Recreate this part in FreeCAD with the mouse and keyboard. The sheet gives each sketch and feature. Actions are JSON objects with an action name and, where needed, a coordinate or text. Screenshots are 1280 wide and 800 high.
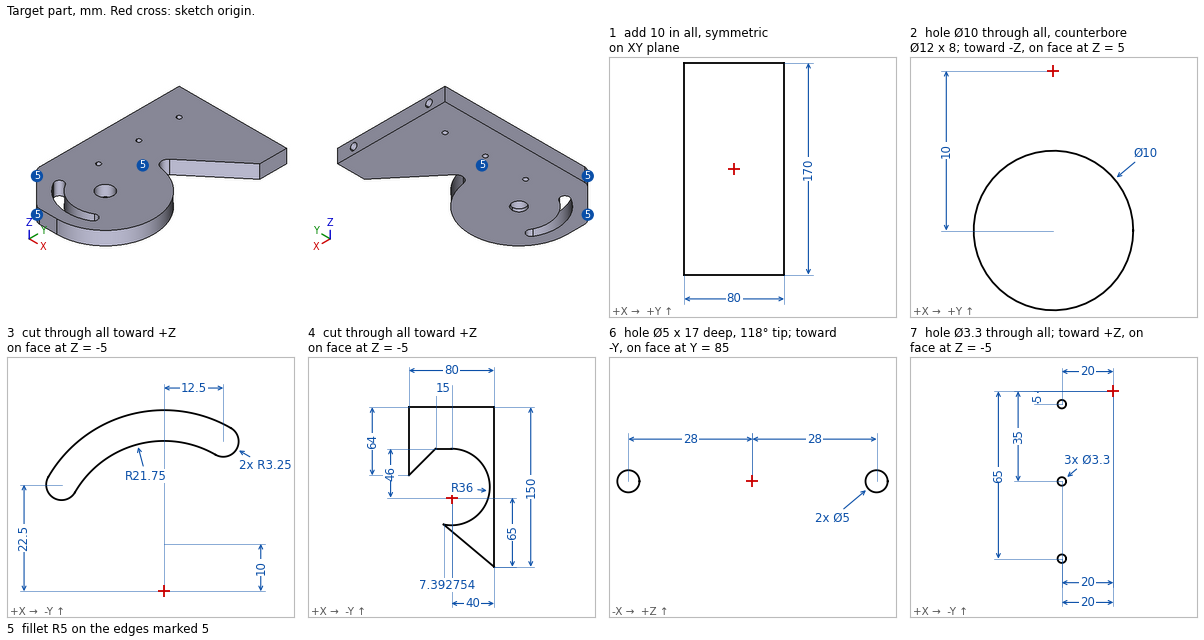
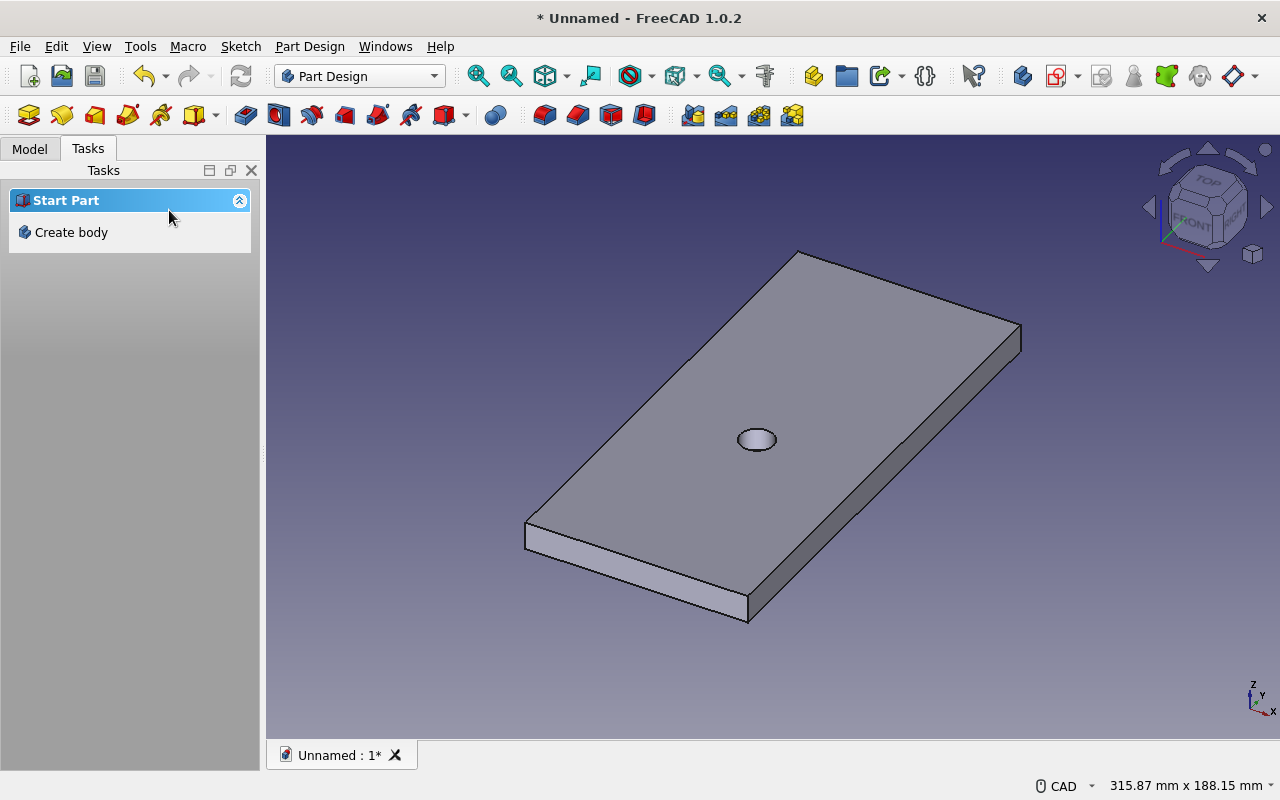
{"action": "key", "text": "5"}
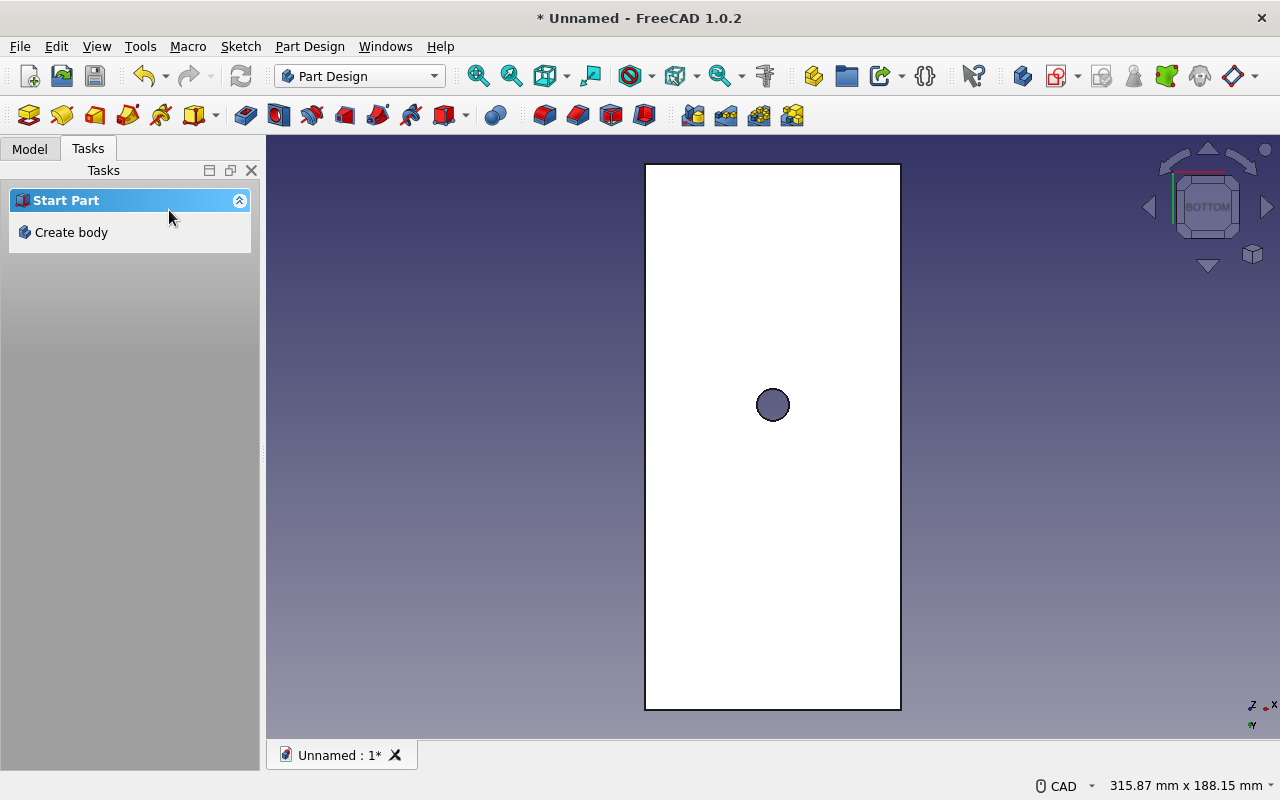
{"action": "left_click", "coordinate": [773, 592]}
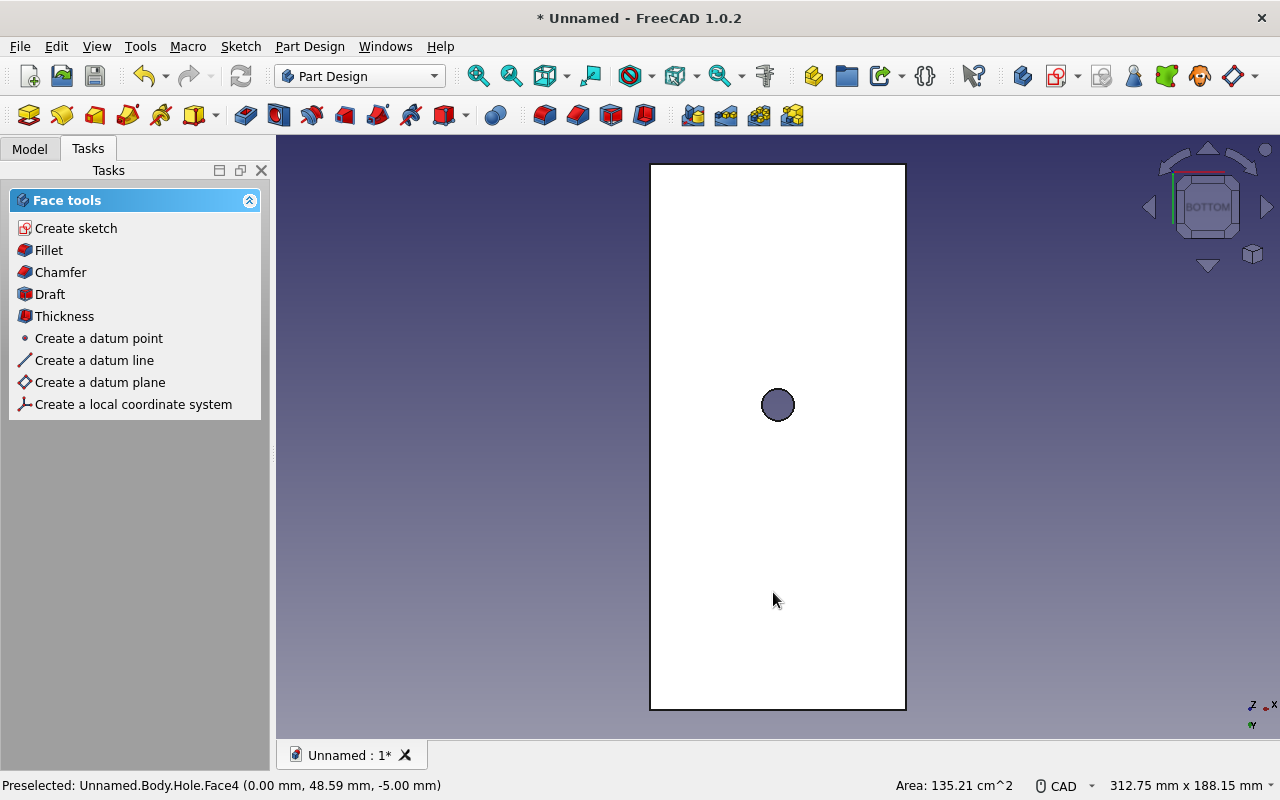
{"action": "left_click", "coordinate": [1056, 76]}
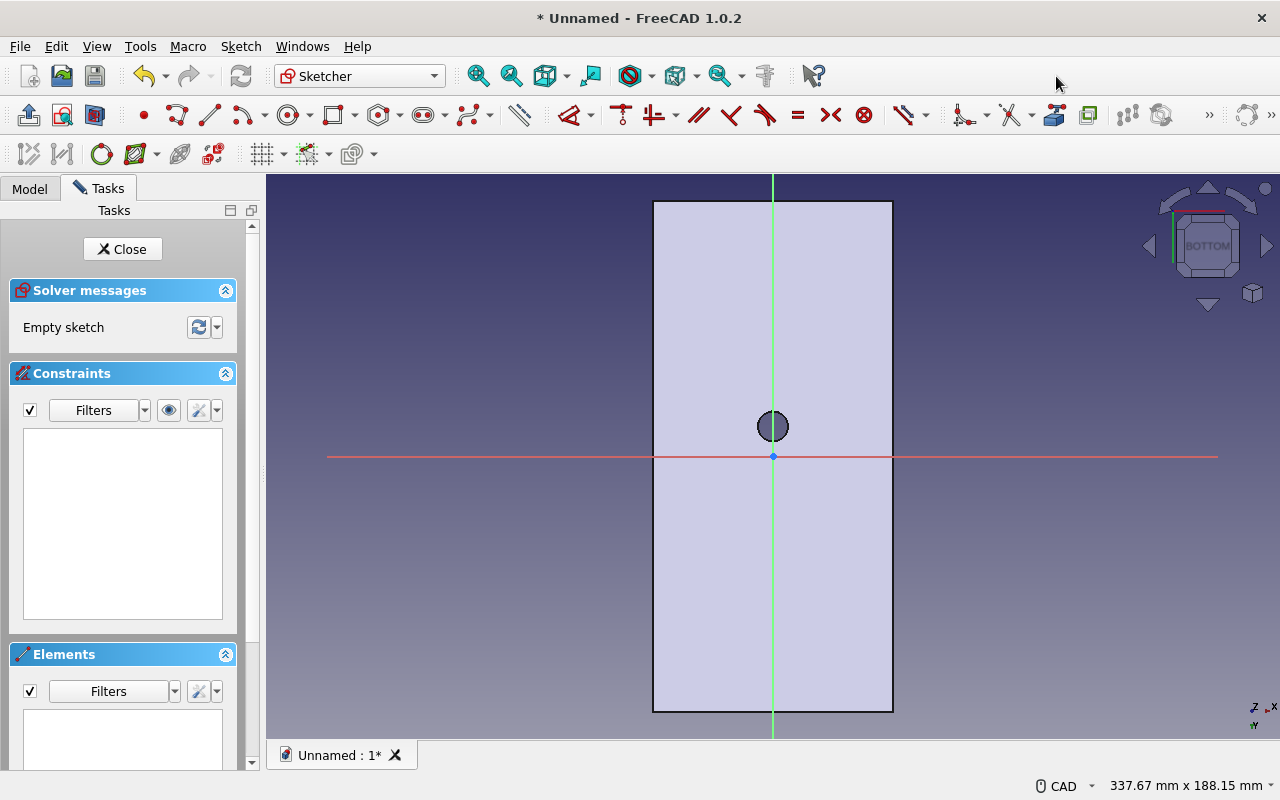
{"action": "scroll", "coordinate": [783, 376], "scroll_direction": "up", "scroll_amount": 6}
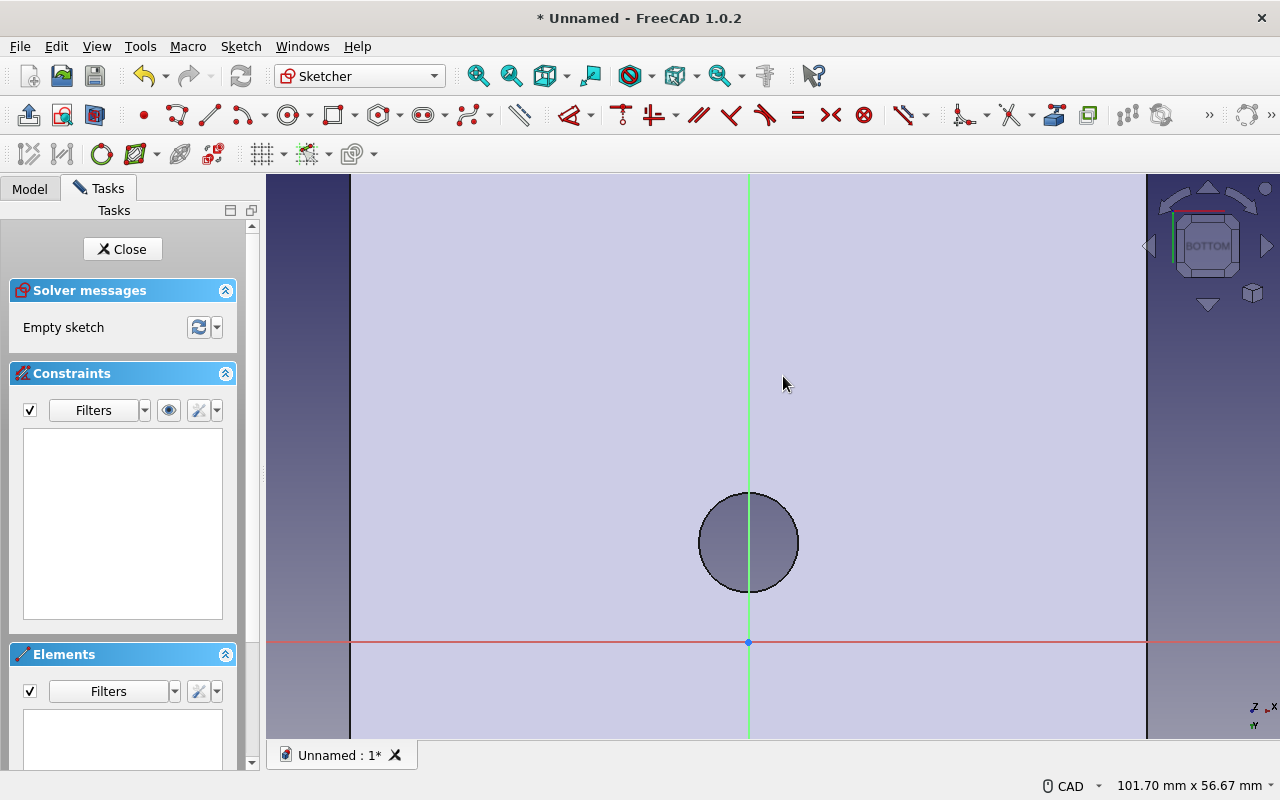
{"action": "key", "text": "g 3 a"}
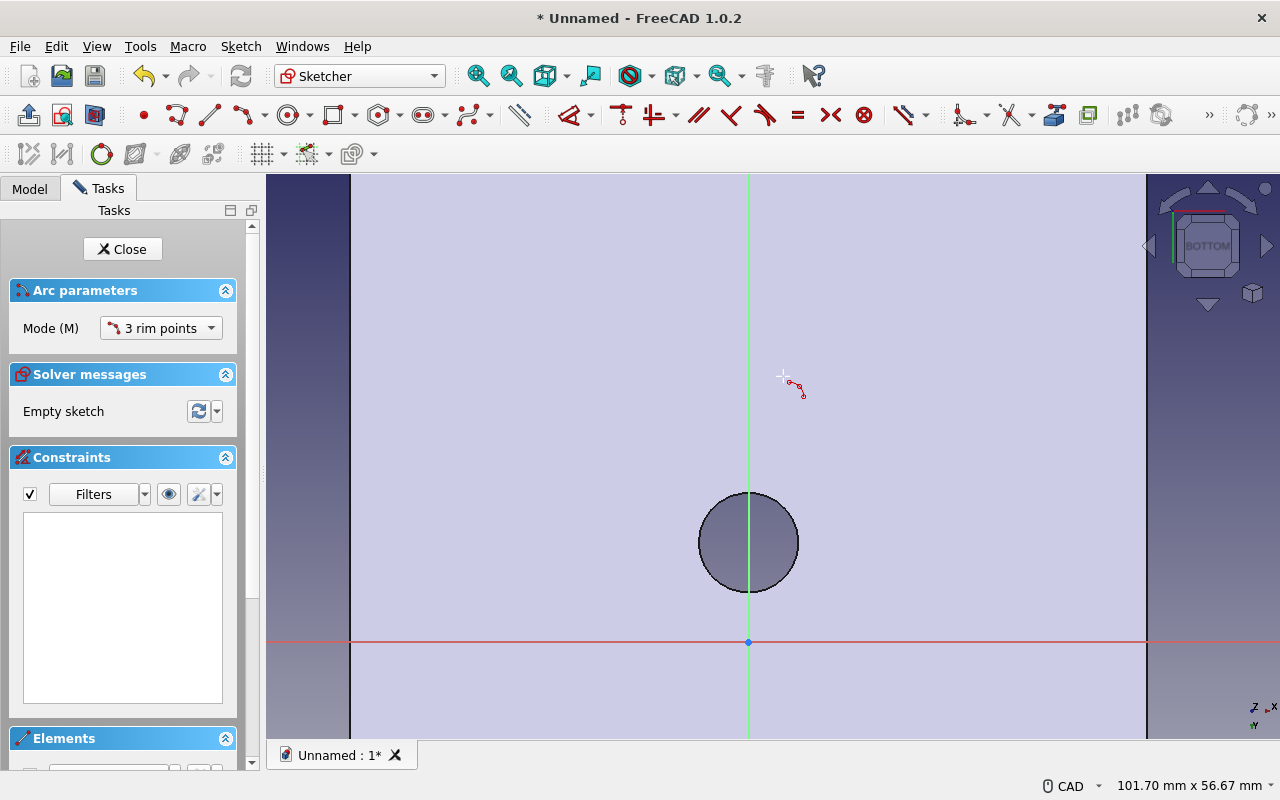
{"action": "left_click", "coordinate": [561, 434]}
{"action": "left_click", "coordinate": [857, 355]}
{"action": "left_click", "coordinate": [692, 333]}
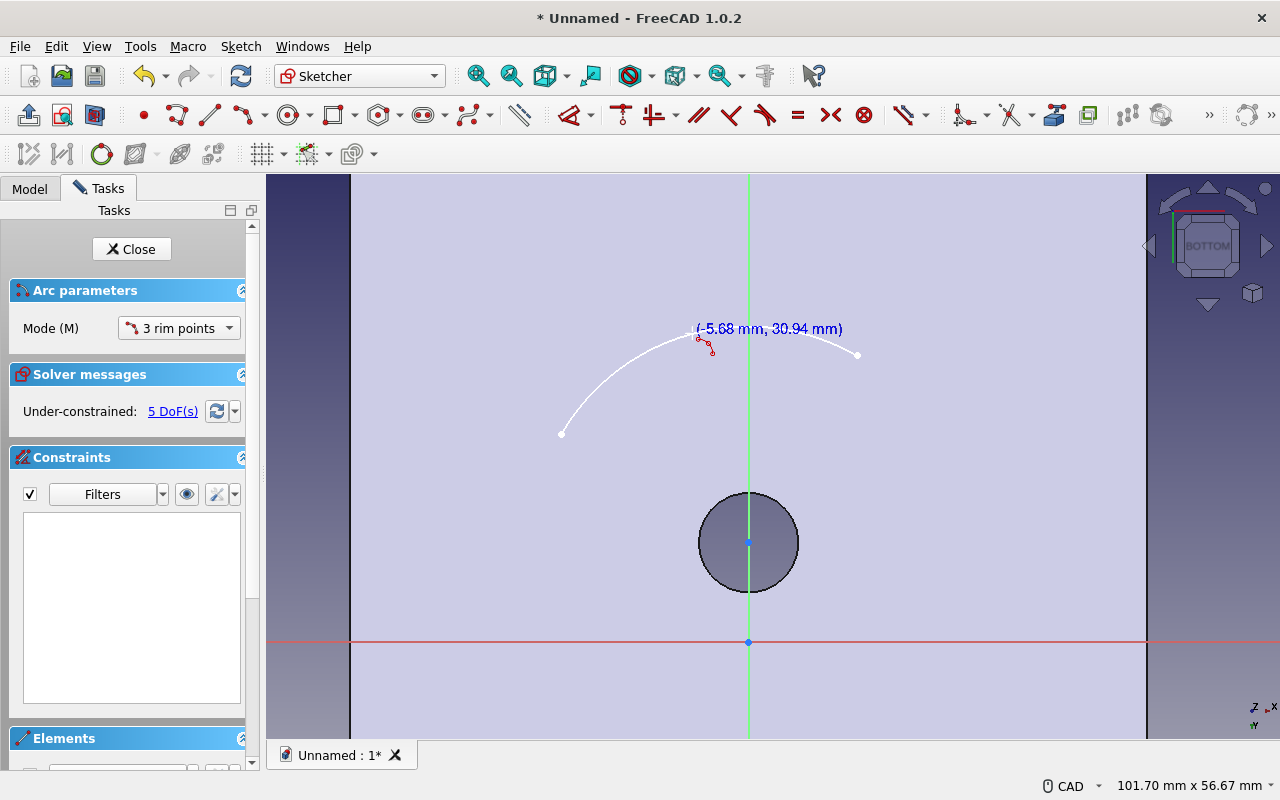
{"action": "left_click", "coordinate": [857, 356]}
{"action": "left_click", "coordinate": [889, 299]}
{"action": "left_click", "coordinate": [901, 343]}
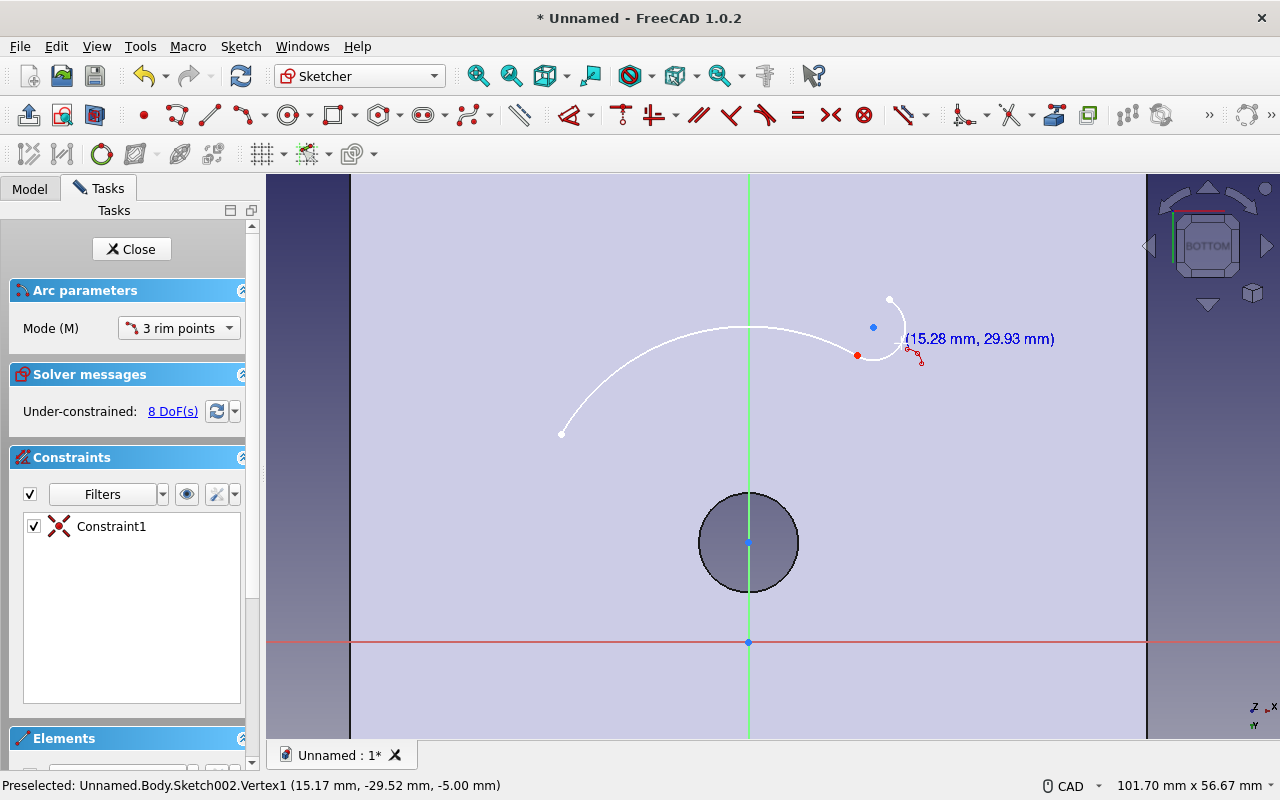
{"action": "left_click", "coordinate": [889, 300]}
{"action": "left_click", "coordinate": [505, 402]}
{"action": "left_click", "coordinate": [676, 271]}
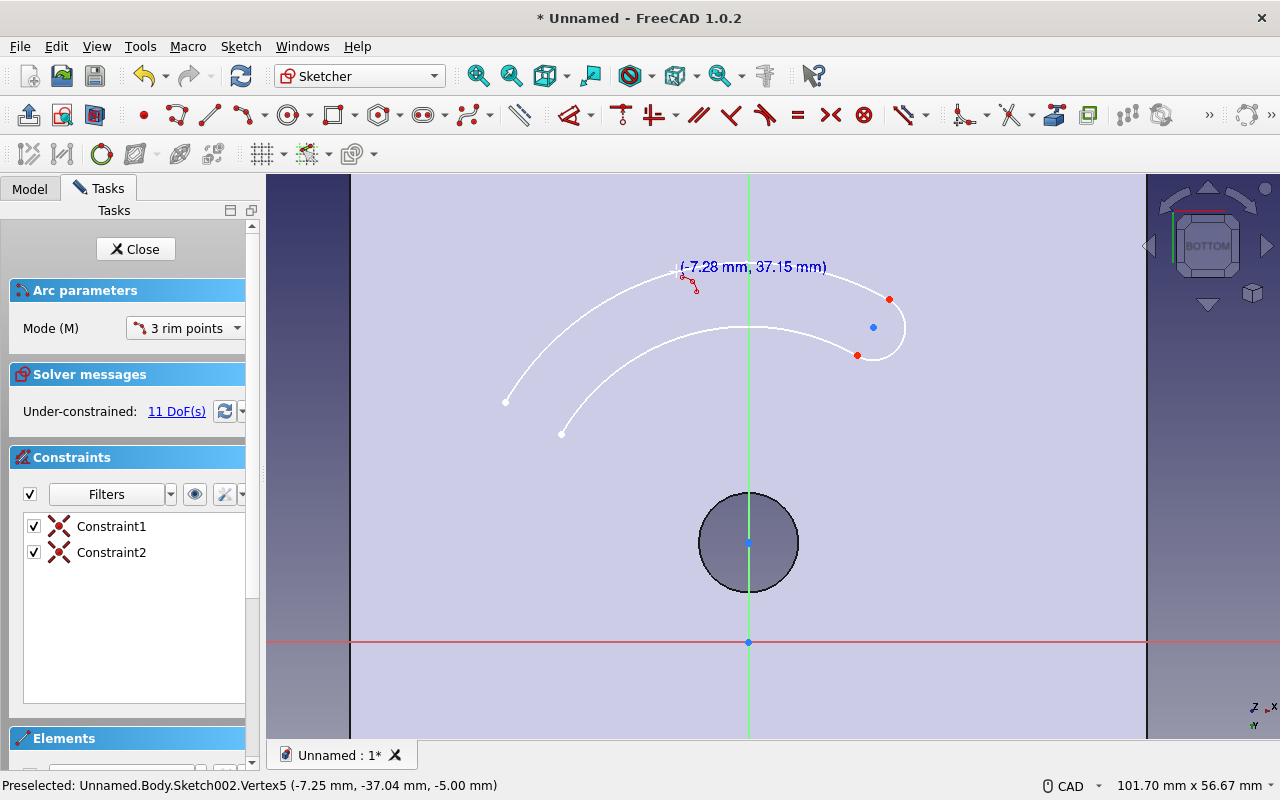
{"action": "left_click", "coordinate": [505, 403]}
{"action": "left_click", "coordinate": [561, 435]}
{"action": "left_click", "coordinate": [517, 446]}
{"action": "key", "text": "Escape"}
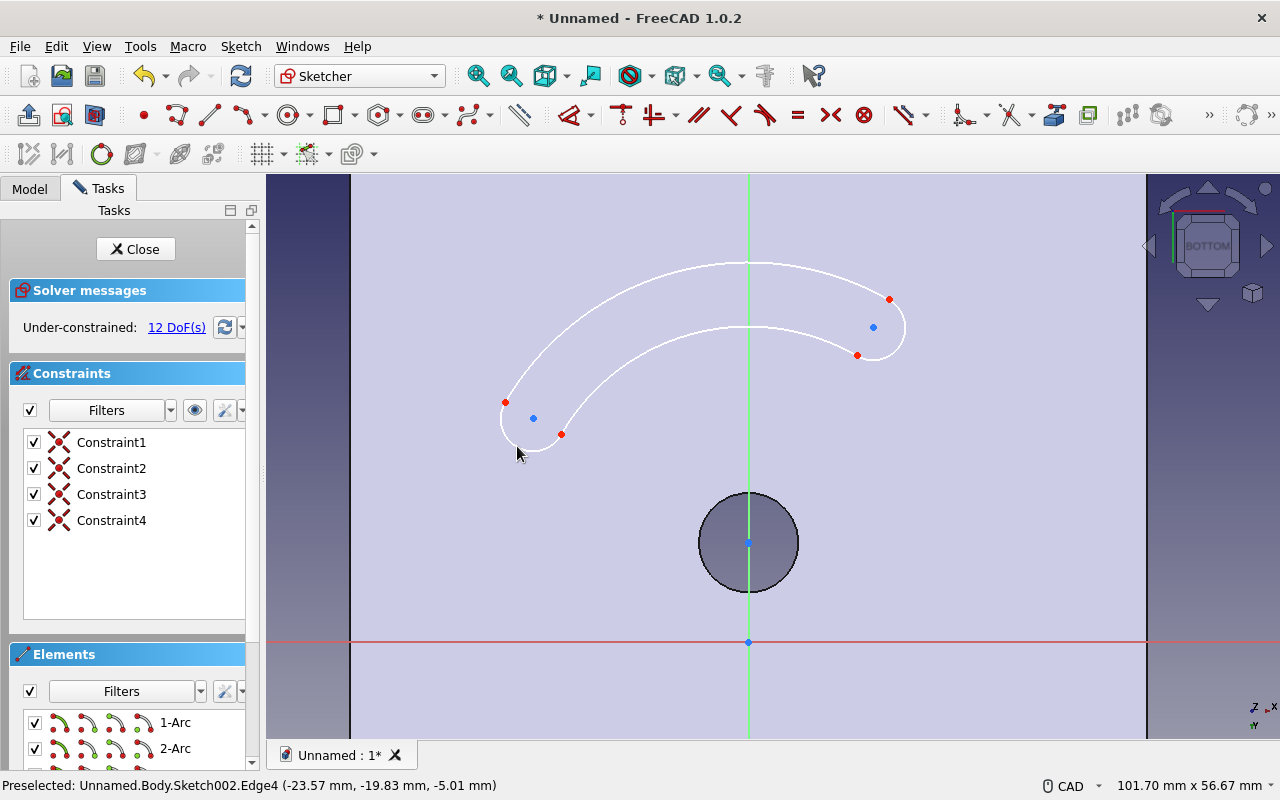
{"action": "left_click", "coordinate": [760, 327]}